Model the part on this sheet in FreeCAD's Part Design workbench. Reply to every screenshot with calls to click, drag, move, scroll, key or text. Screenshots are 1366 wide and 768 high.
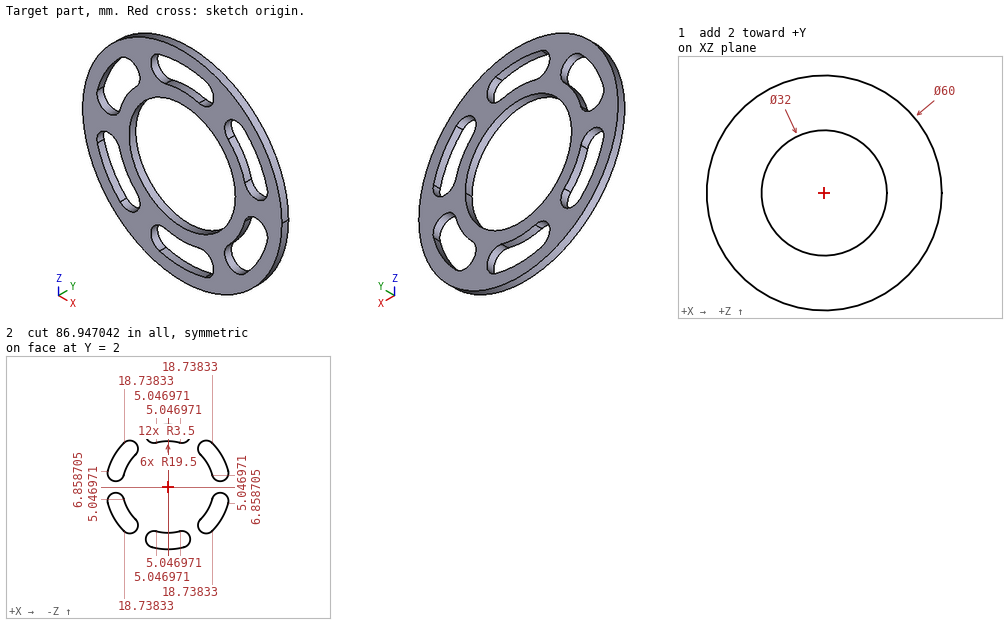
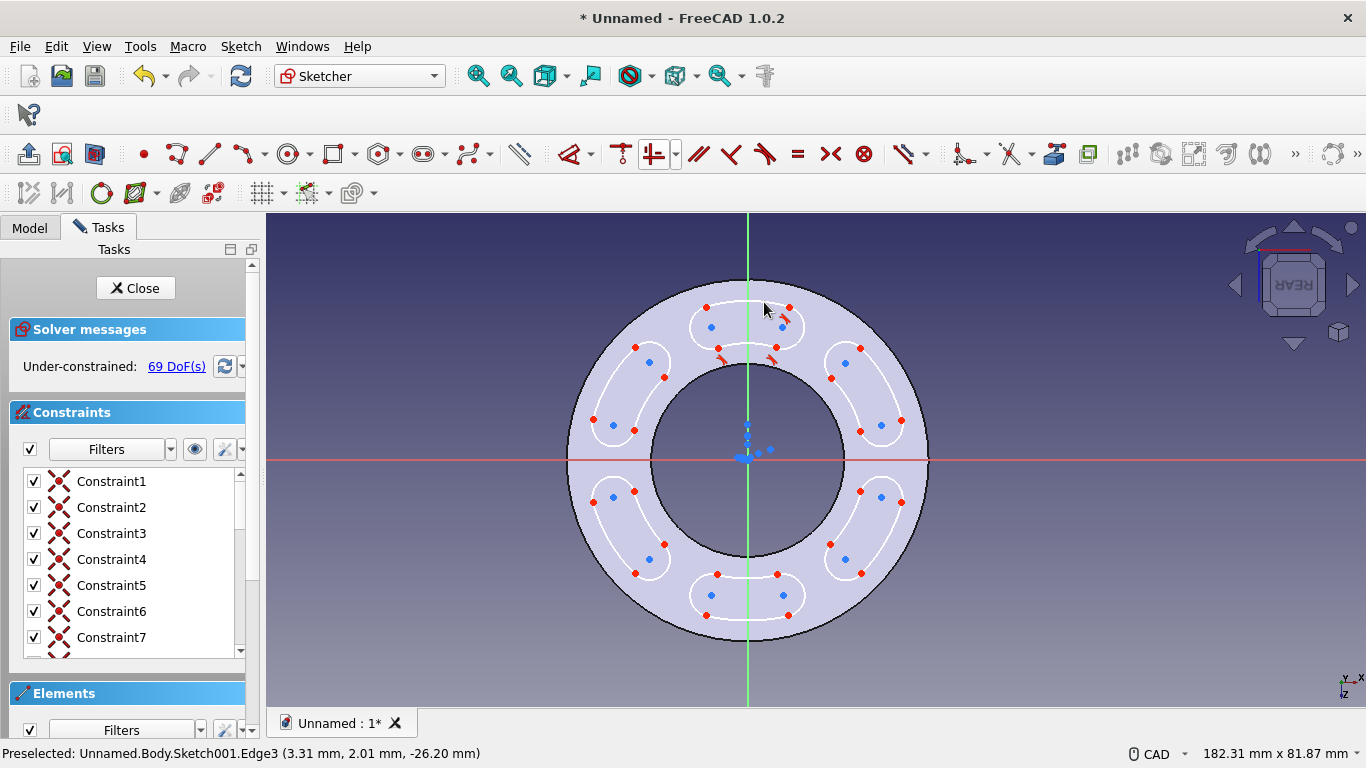
click(764, 302)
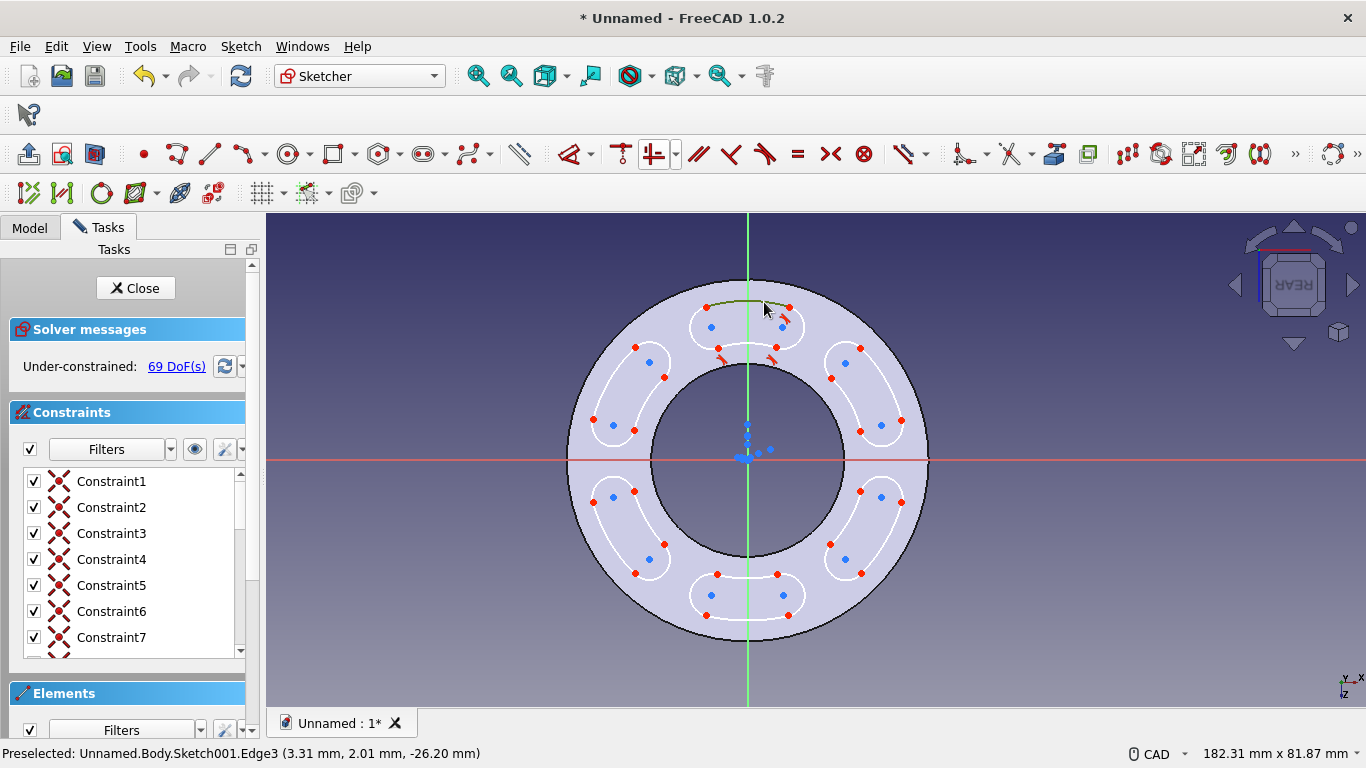
click(691, 320)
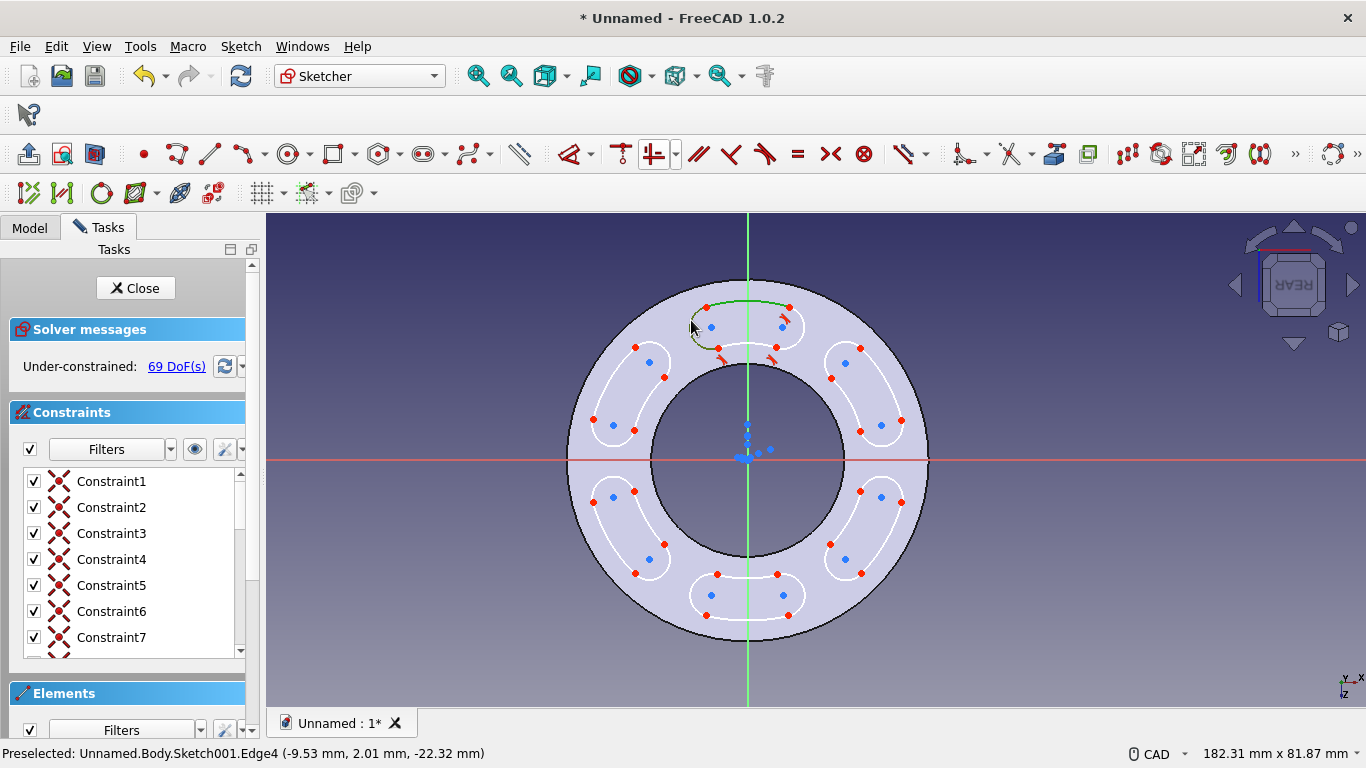
click(765, 154)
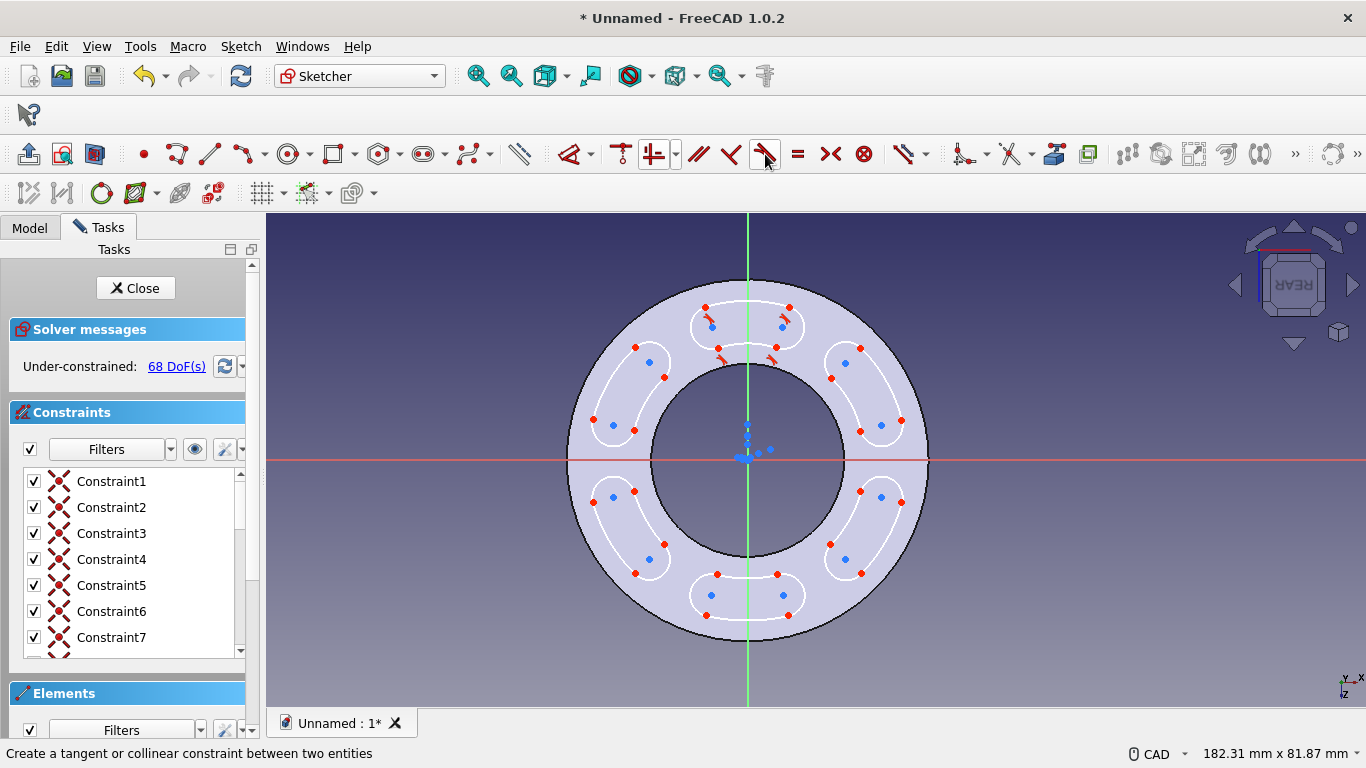
click(855, 413)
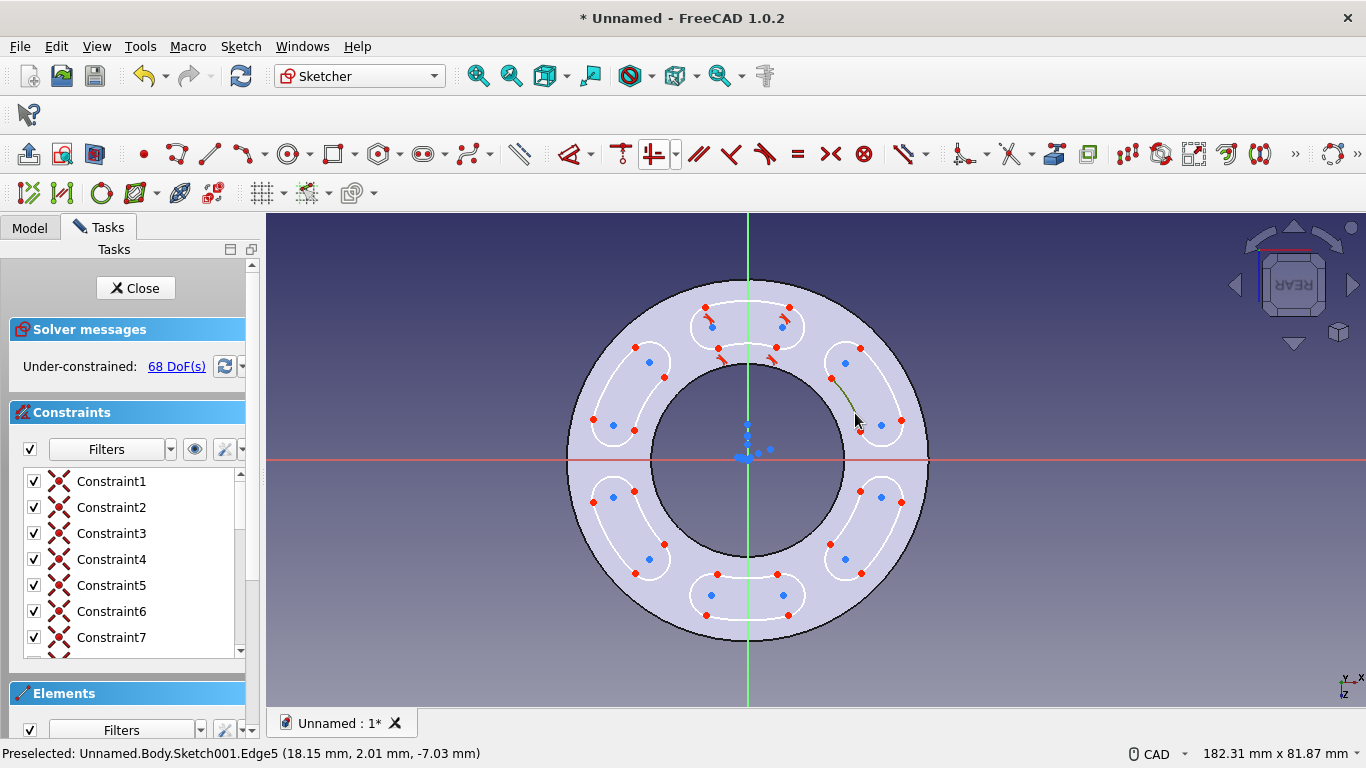
click(874, 445)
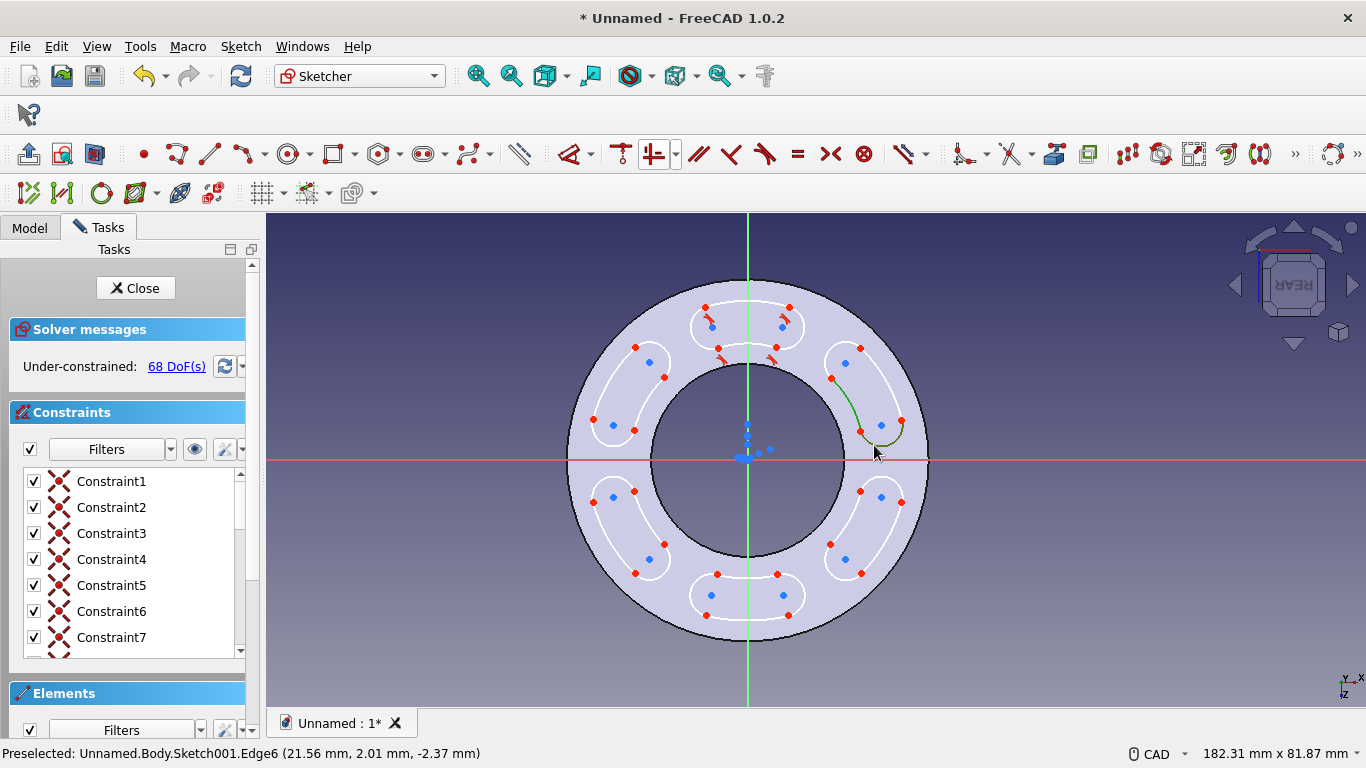
click(765, 154)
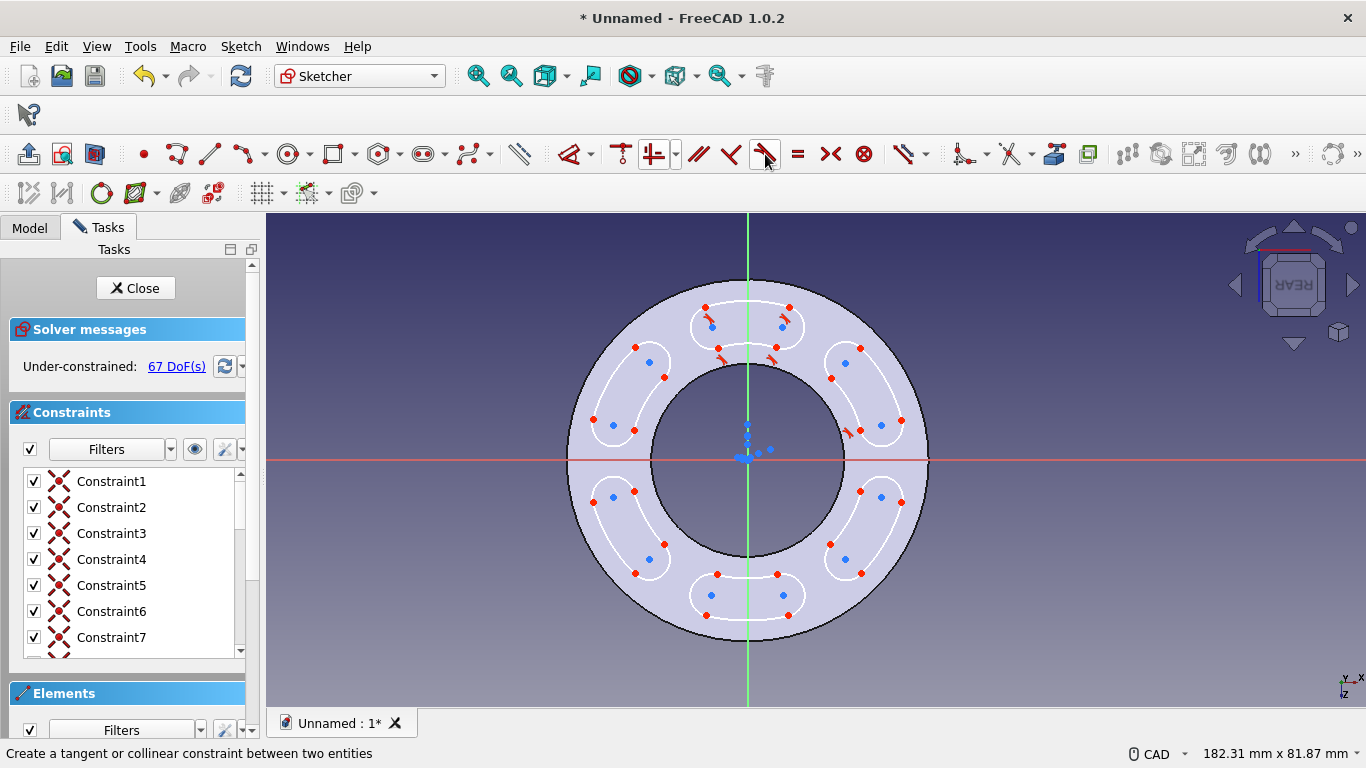
click(855, 413)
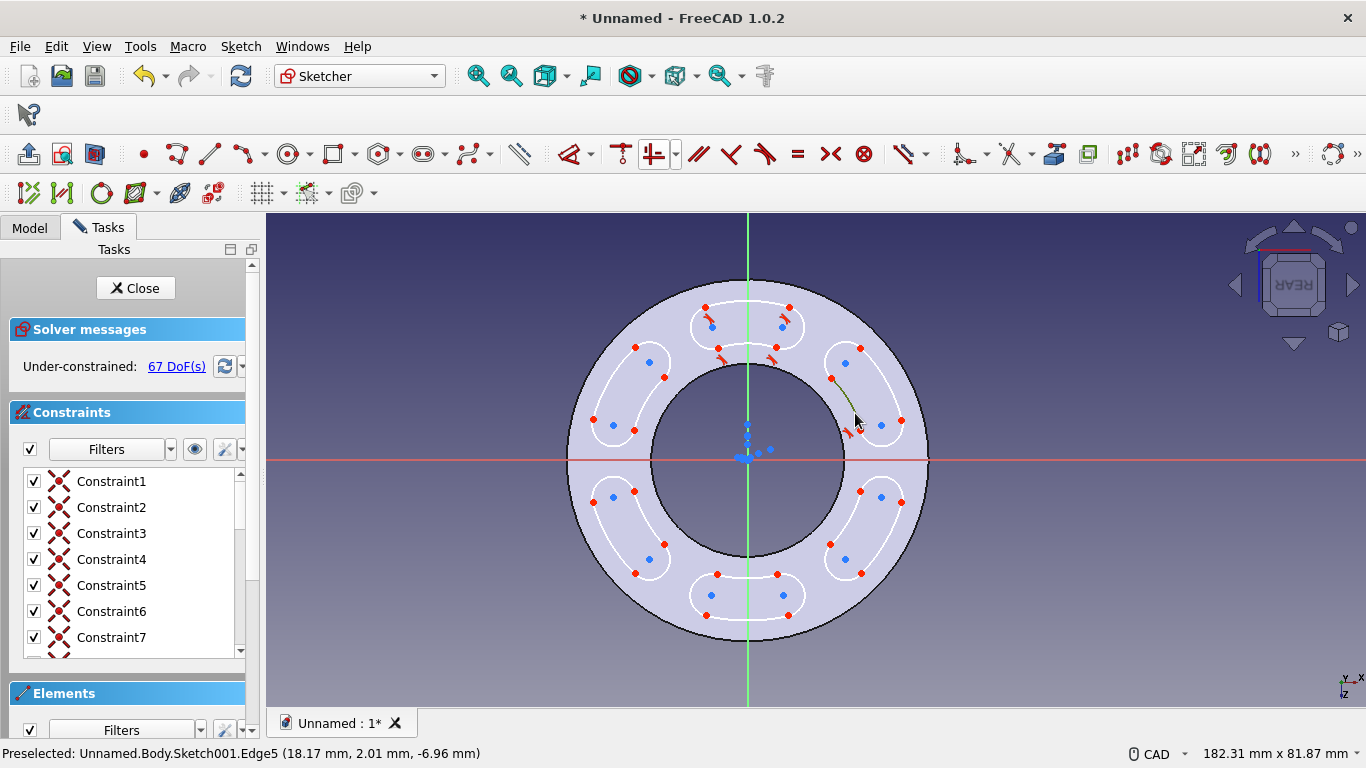
click(843, 342)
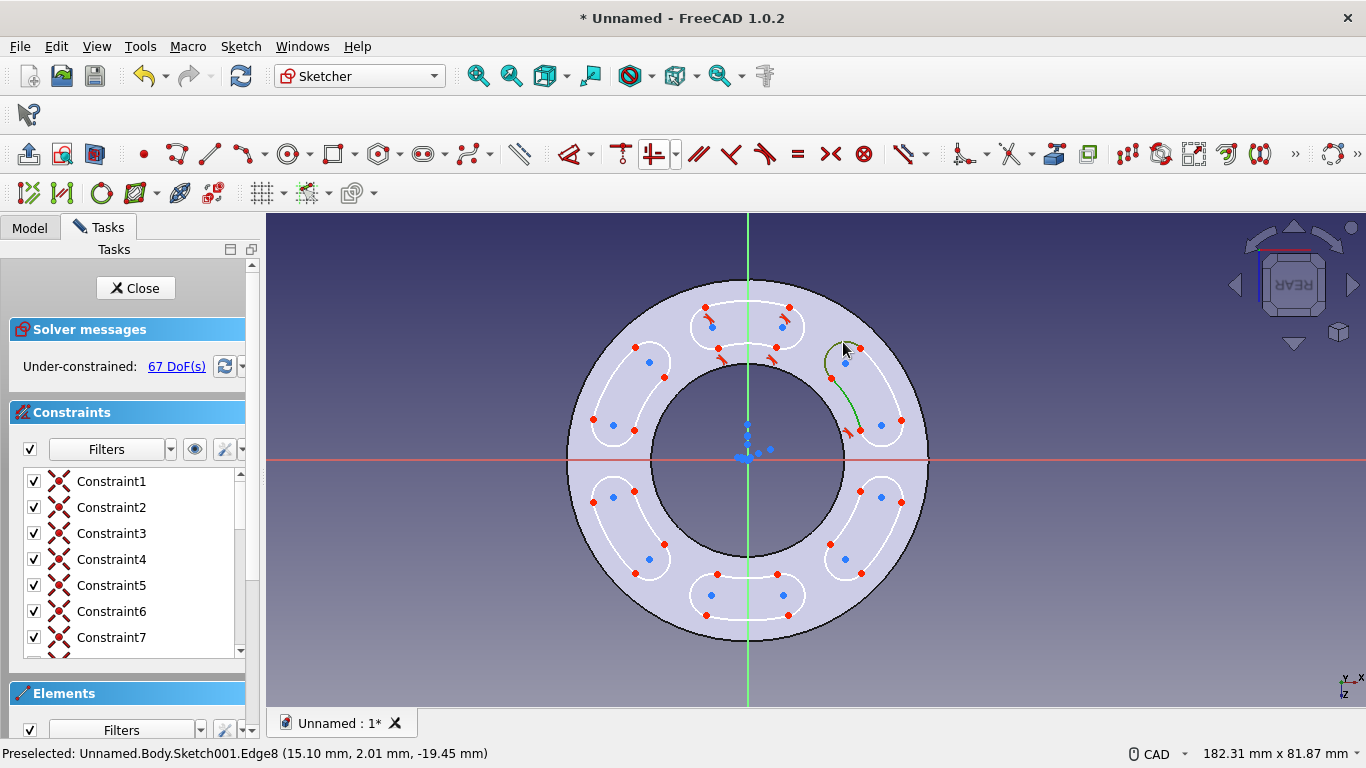
key(t)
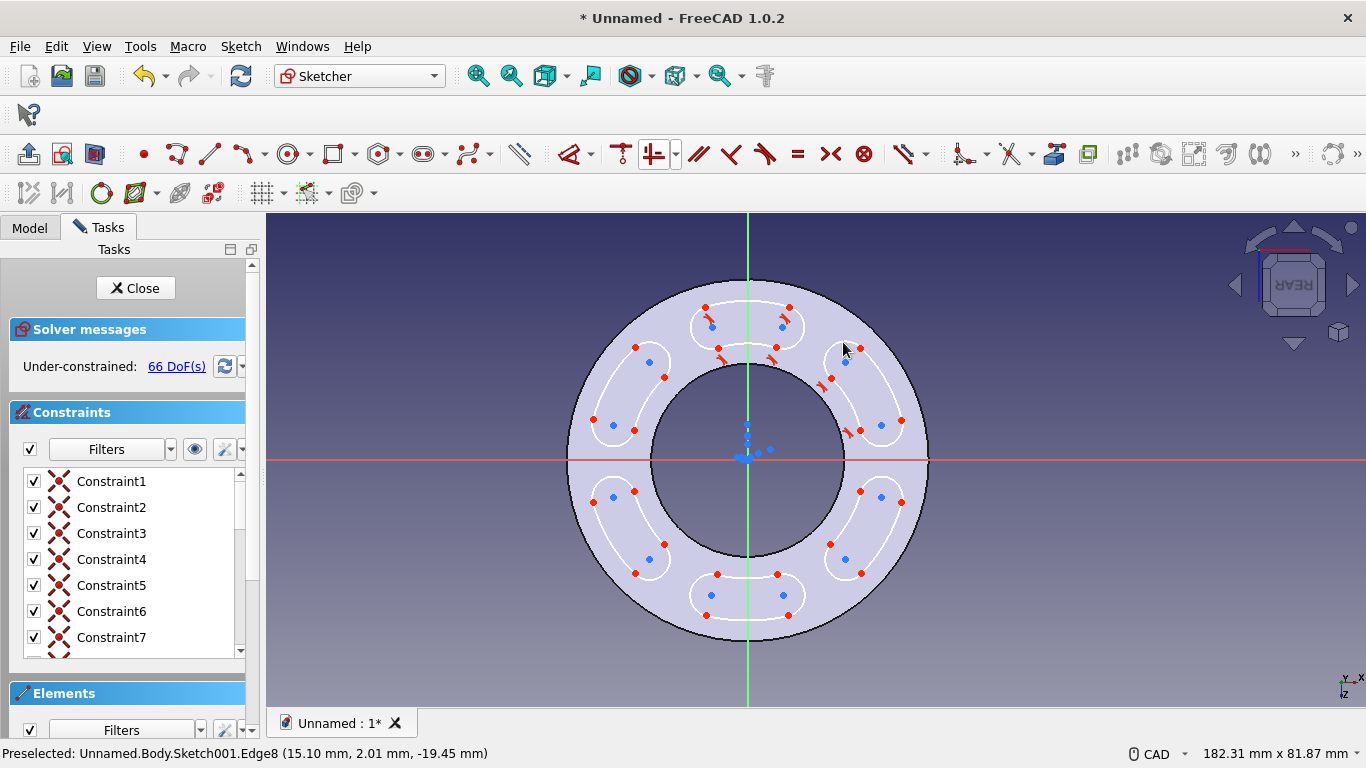
click(873, 445)